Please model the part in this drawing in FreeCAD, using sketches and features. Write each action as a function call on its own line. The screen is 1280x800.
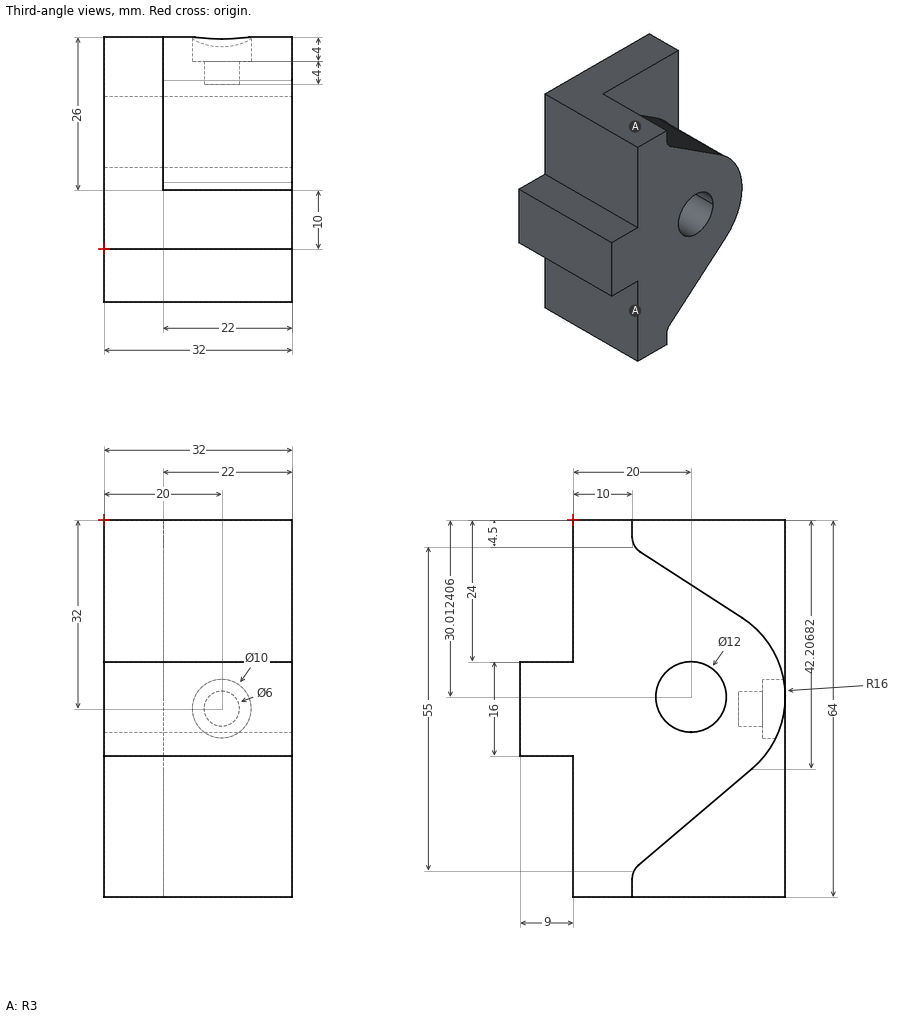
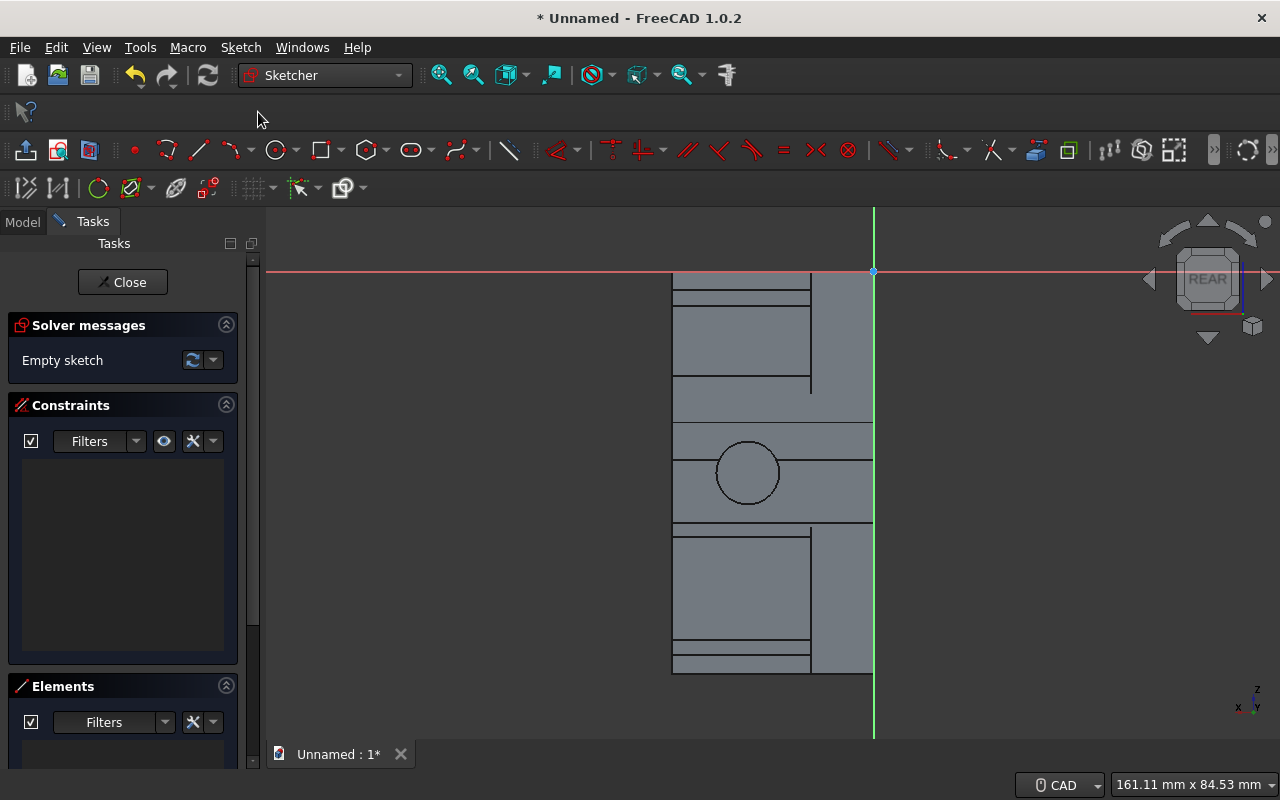
scroll(753, 473, up, 11)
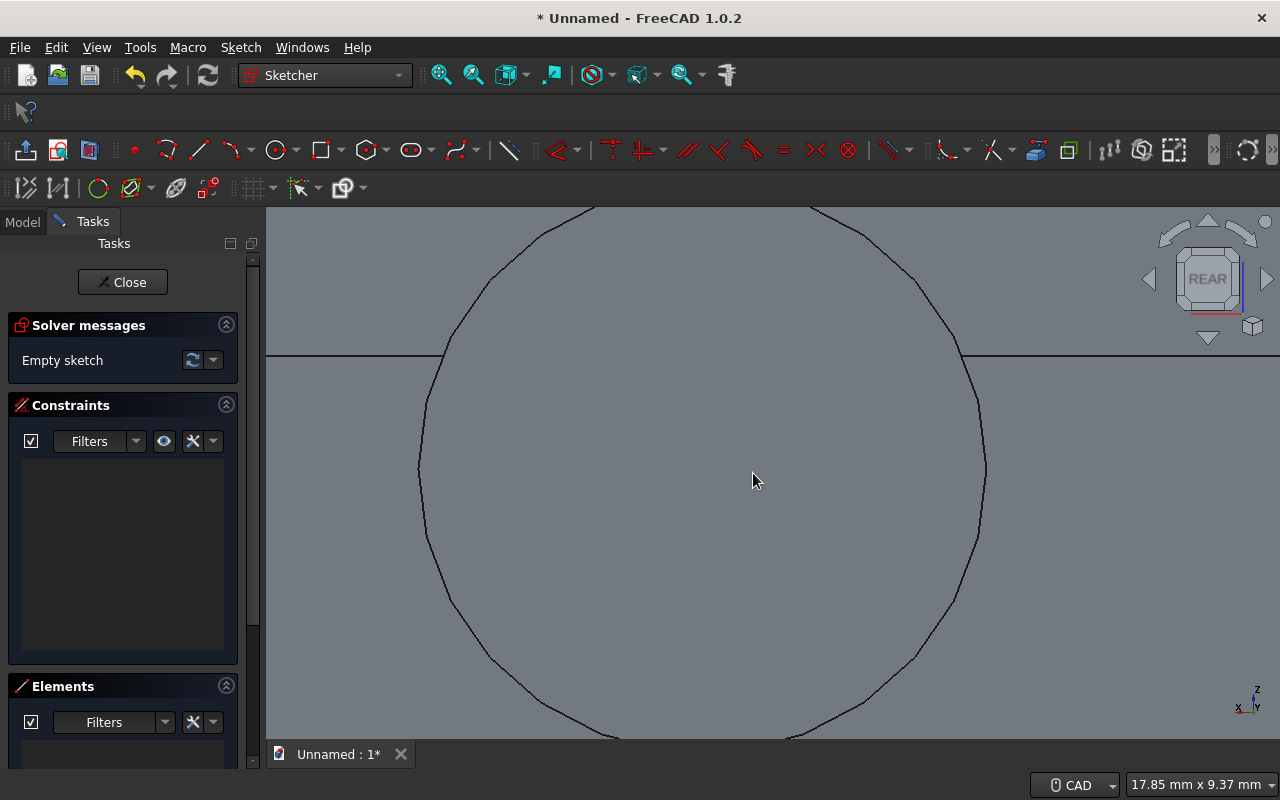
key(g)
key(c)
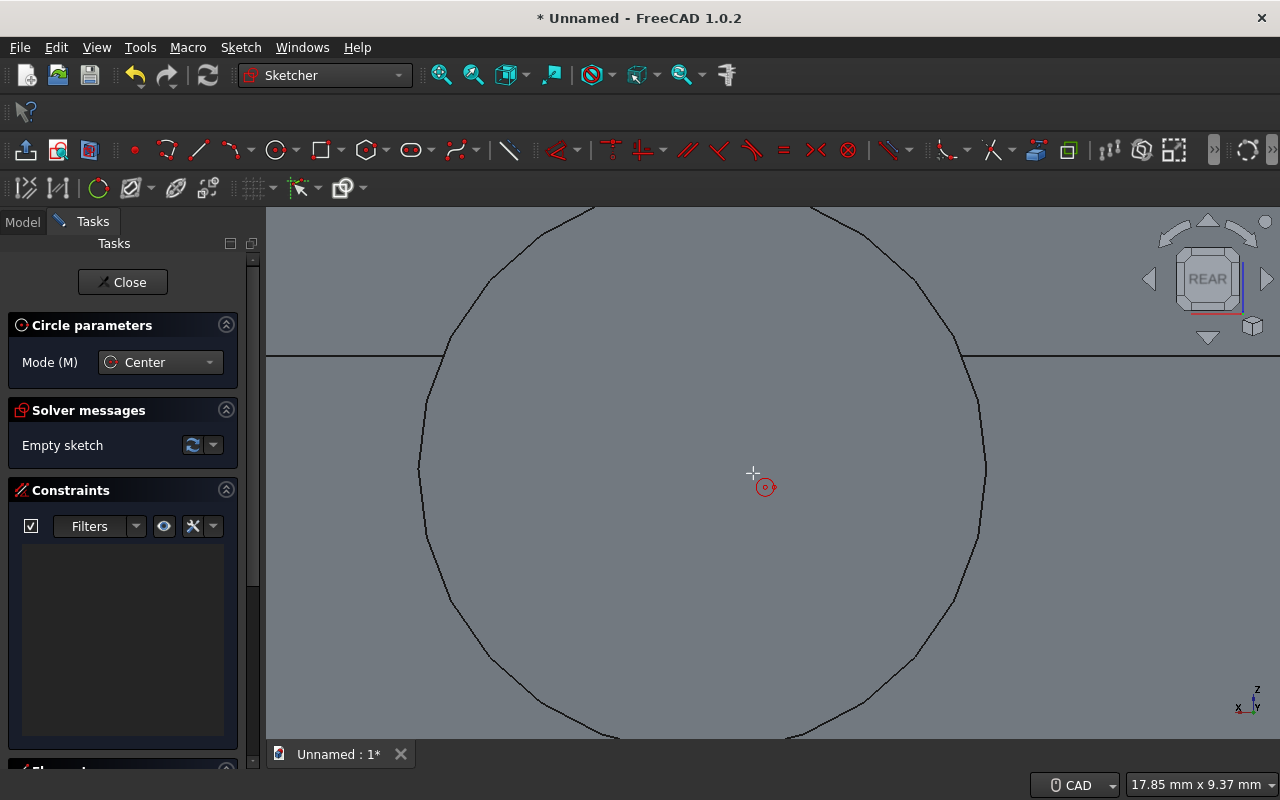
click(702, 469)
move(823, 348)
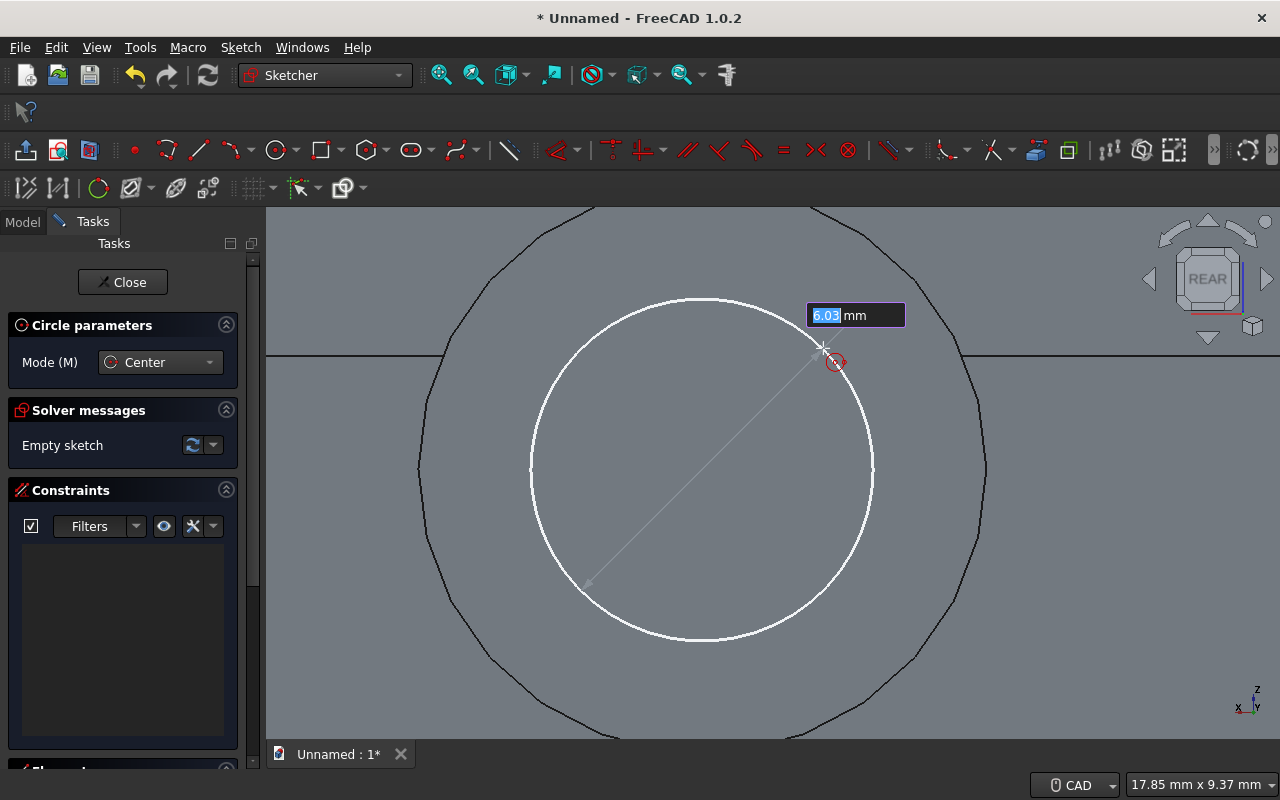
text(6)
key(Return)
key(Escape)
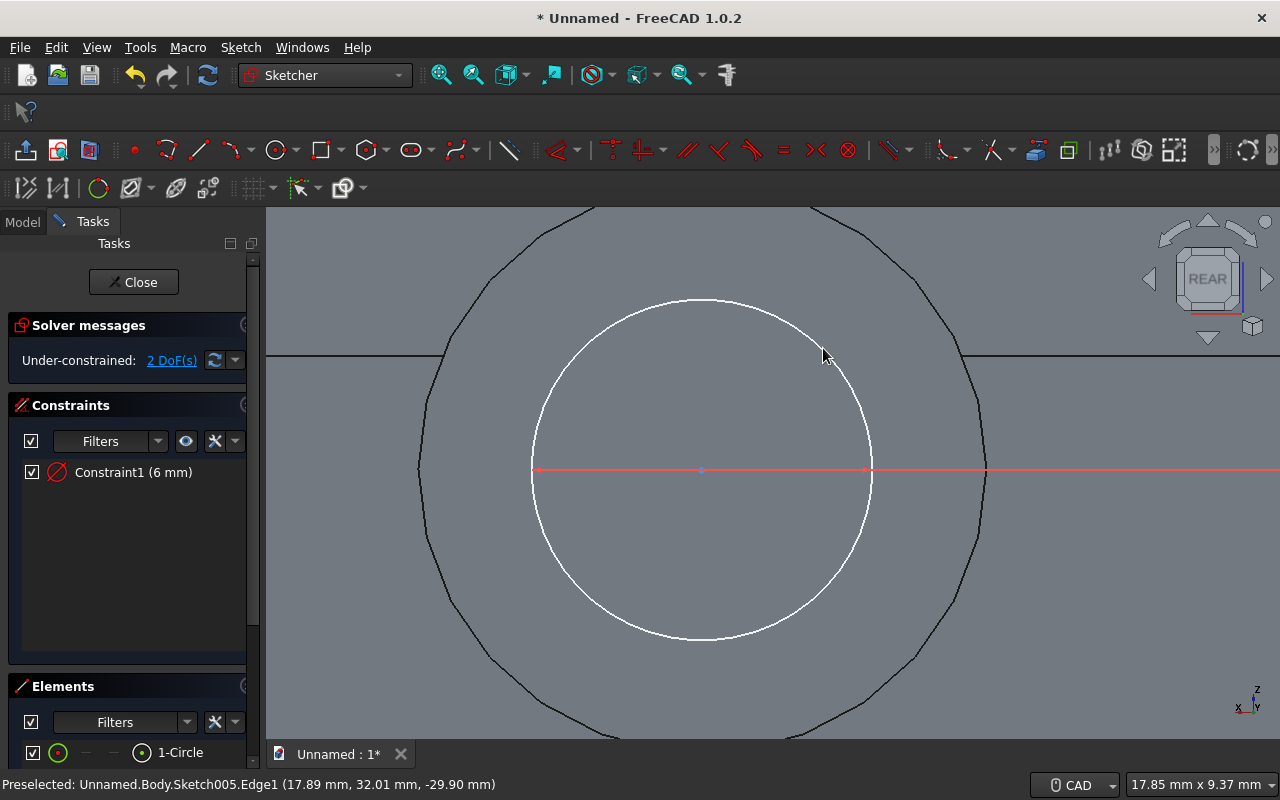
click(556, 150)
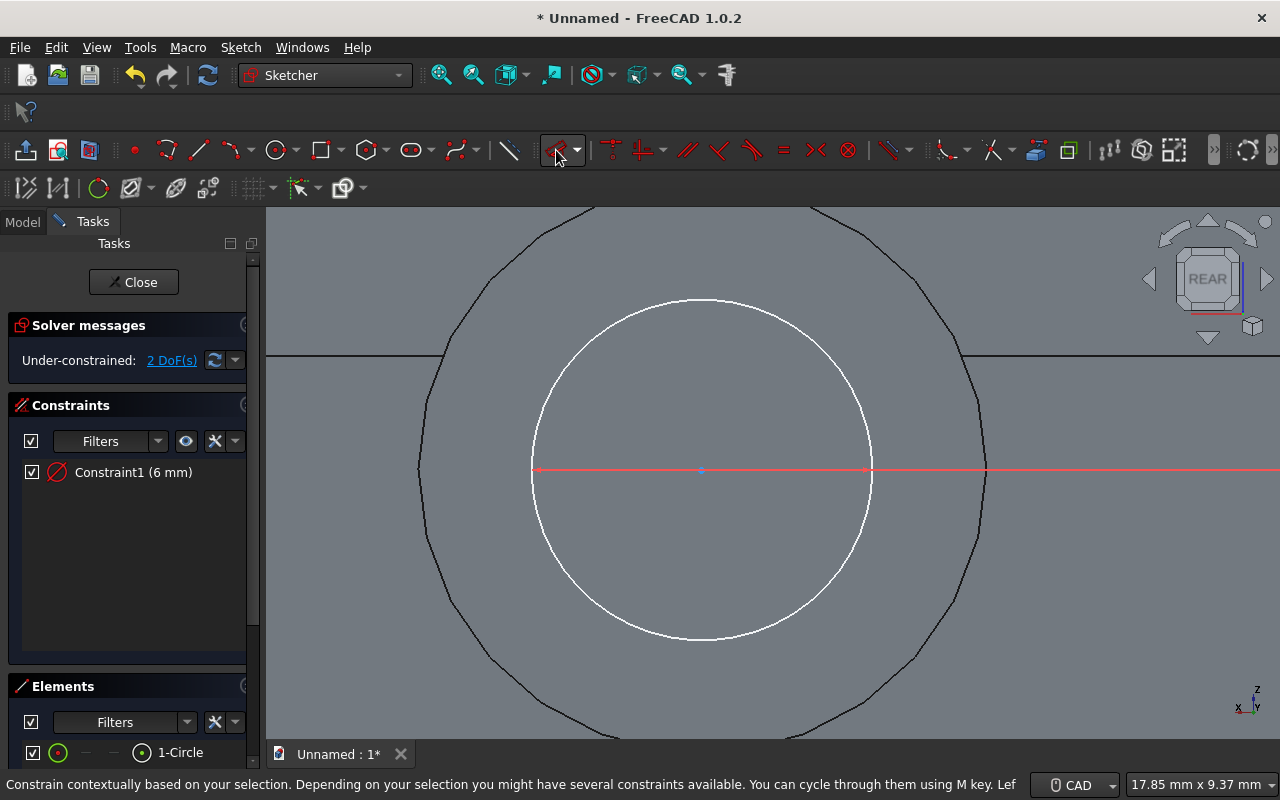
click(702, 470)
click(909, 504)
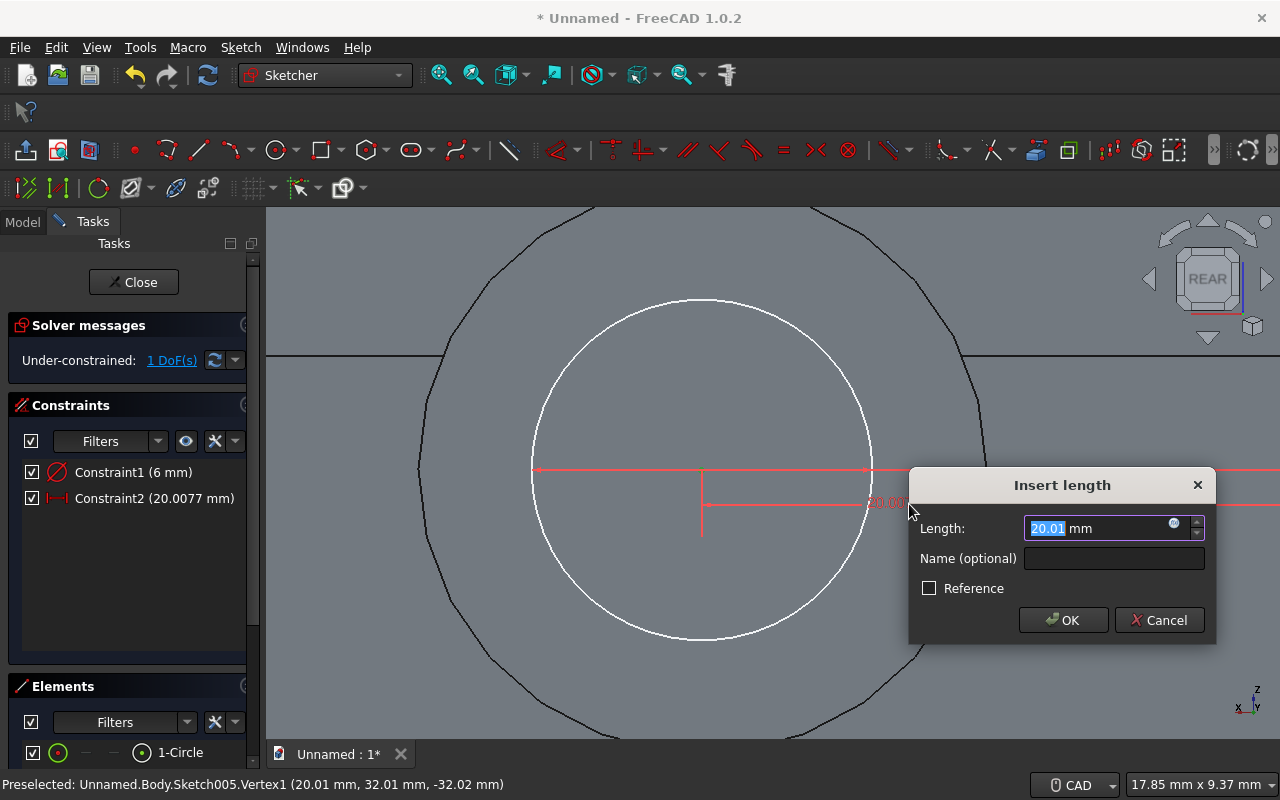
text(20)
key(Return)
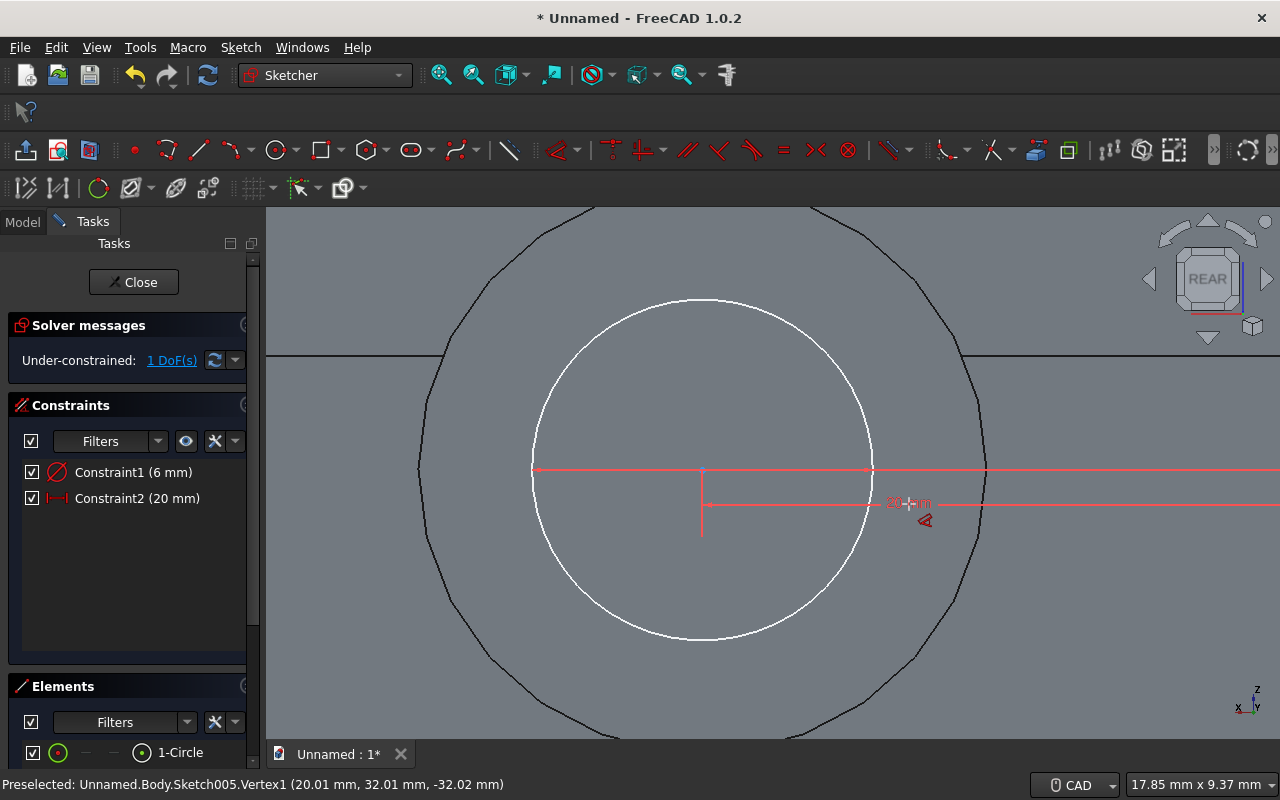
click(702, 470)
click(668, 353)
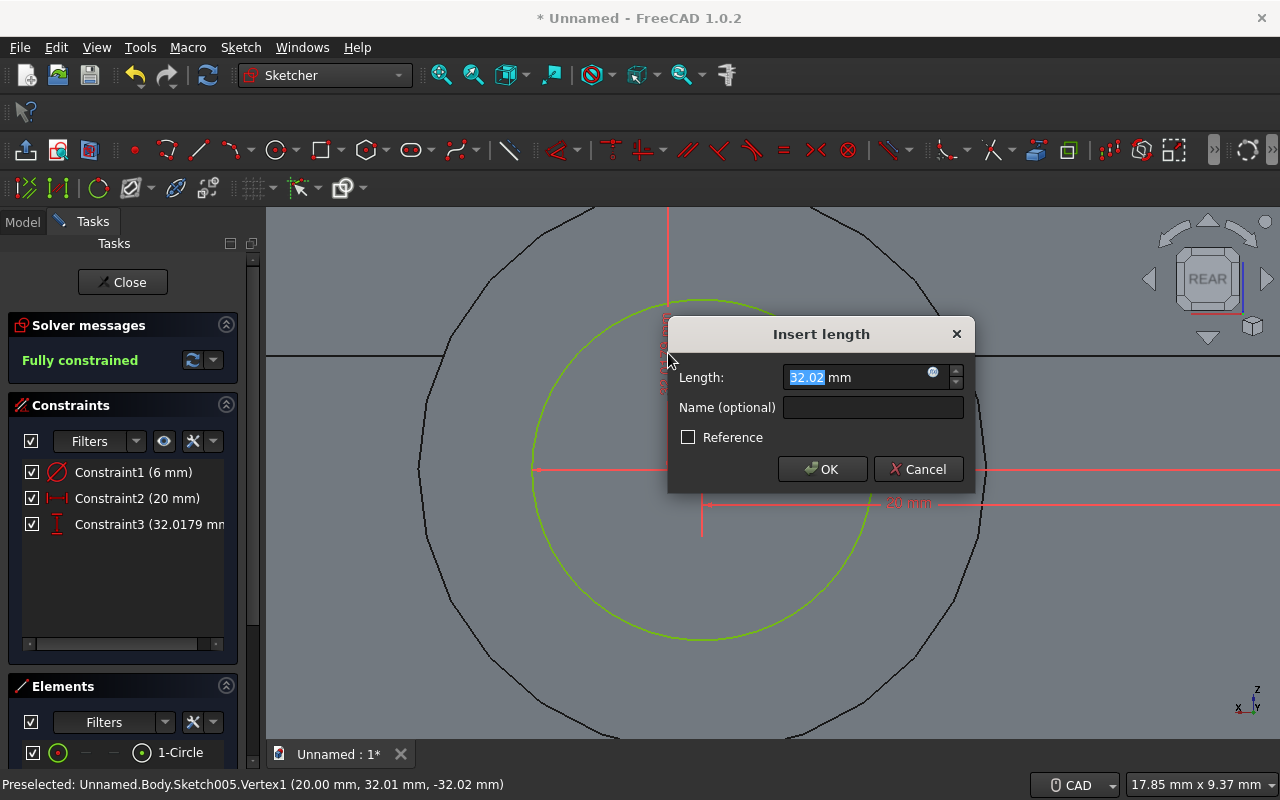
text(32)
key(Return)
key(Escape)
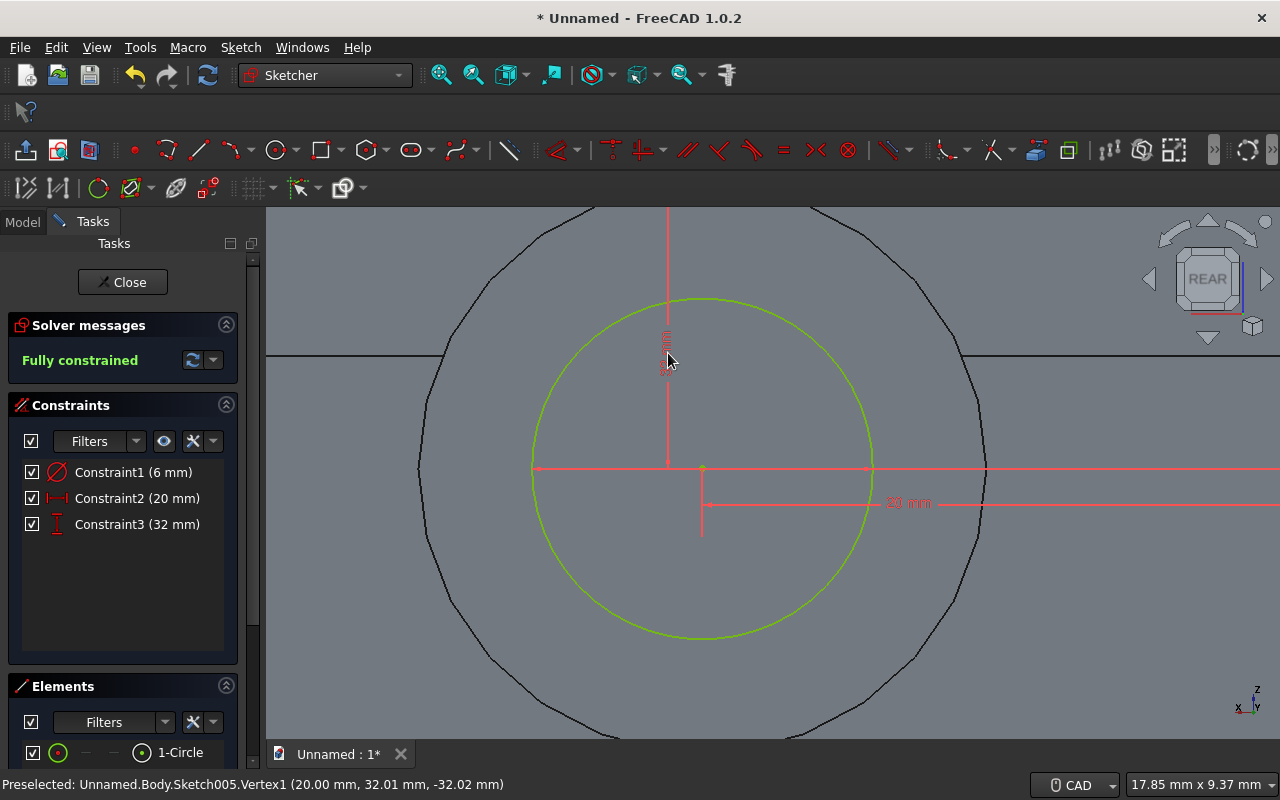
click(123, 282)